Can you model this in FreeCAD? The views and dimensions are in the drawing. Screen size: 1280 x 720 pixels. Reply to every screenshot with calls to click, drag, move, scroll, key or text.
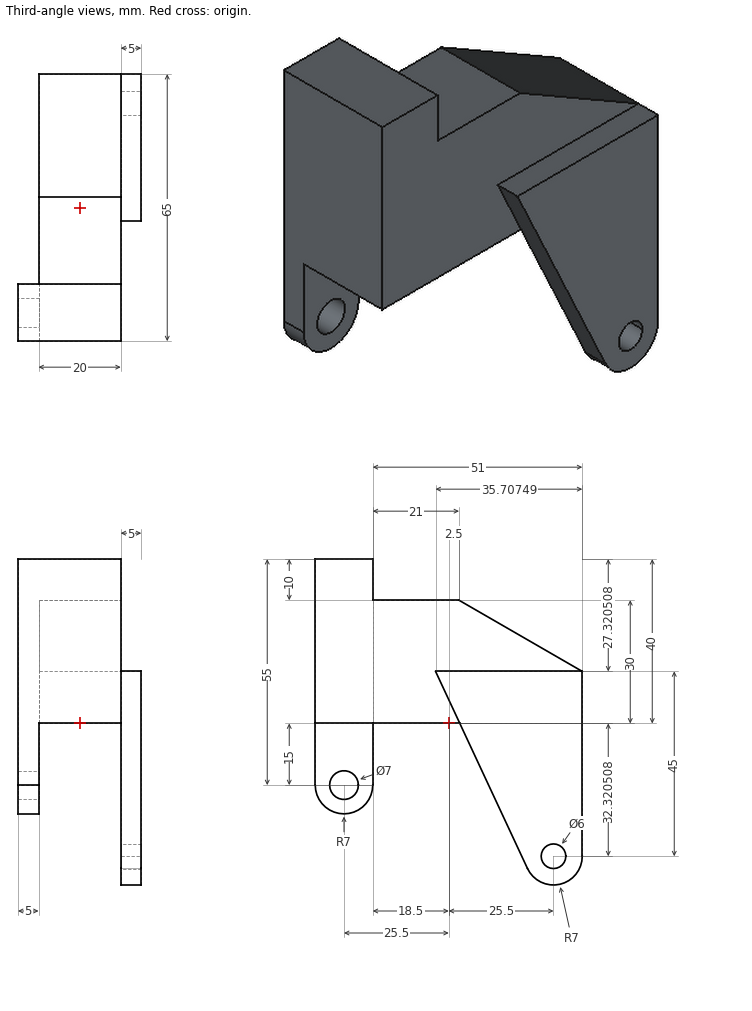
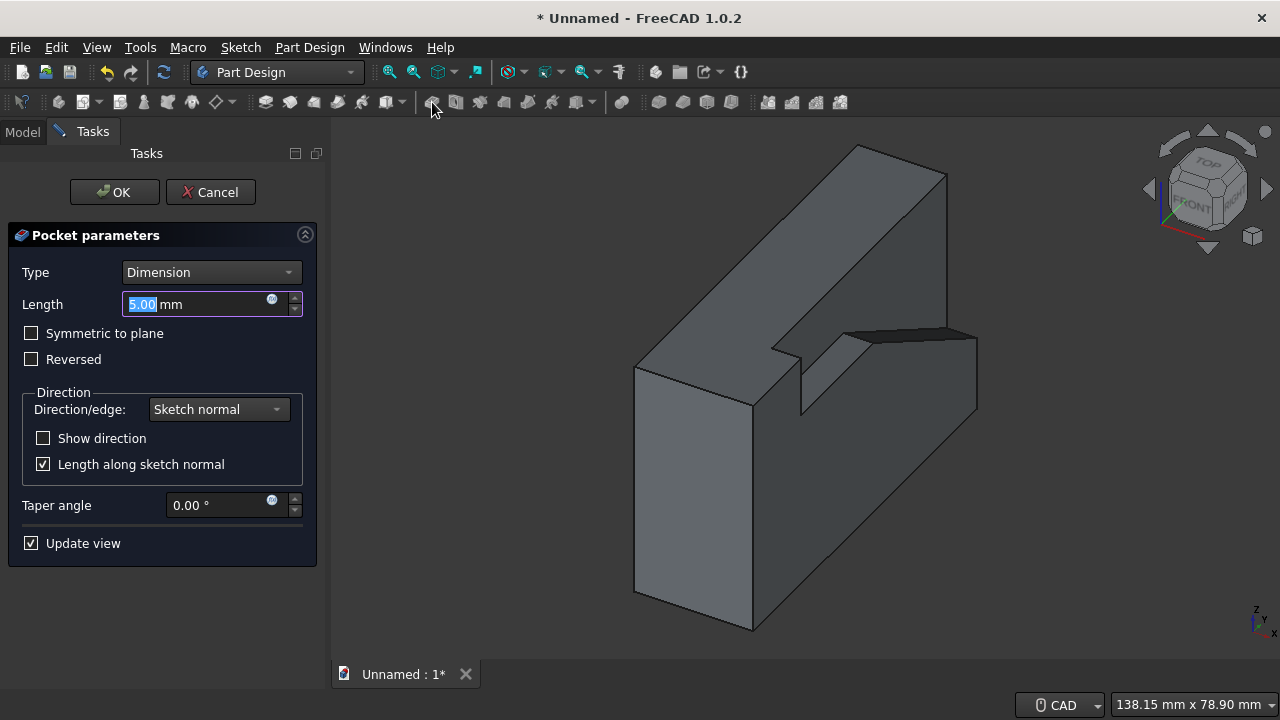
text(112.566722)
key(Tab)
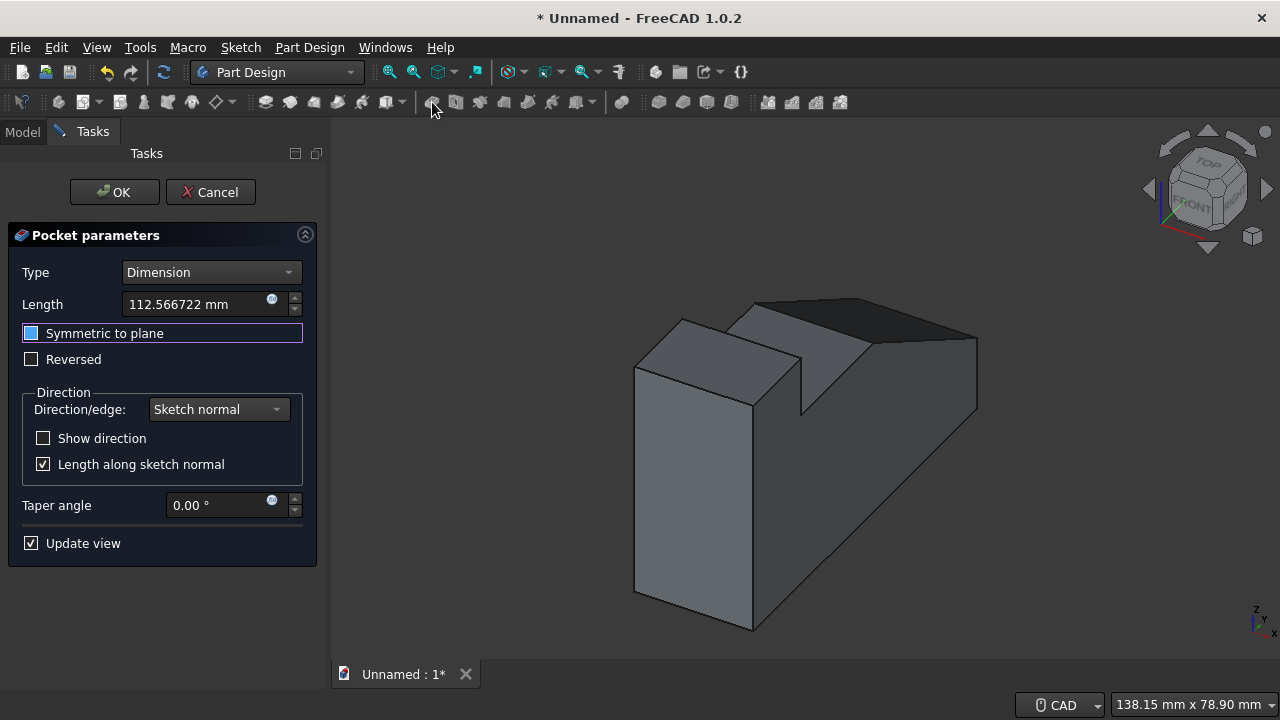
click(30, 333)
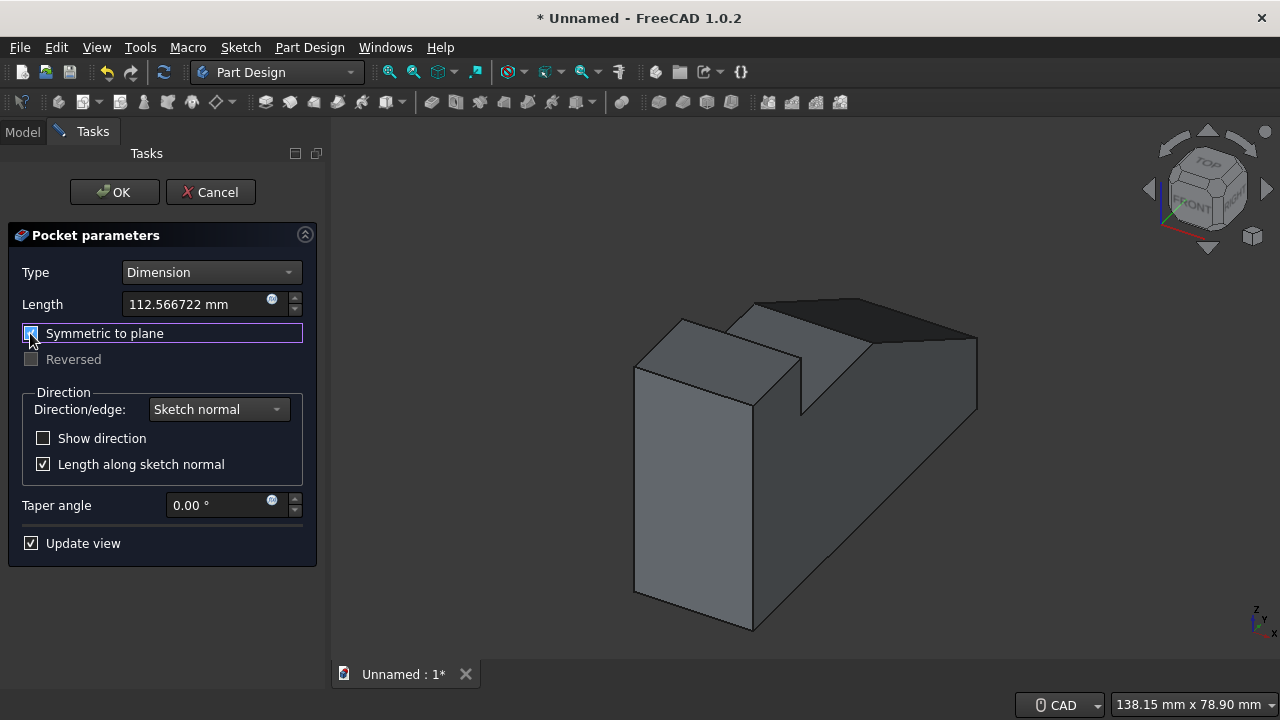
click(115, 192)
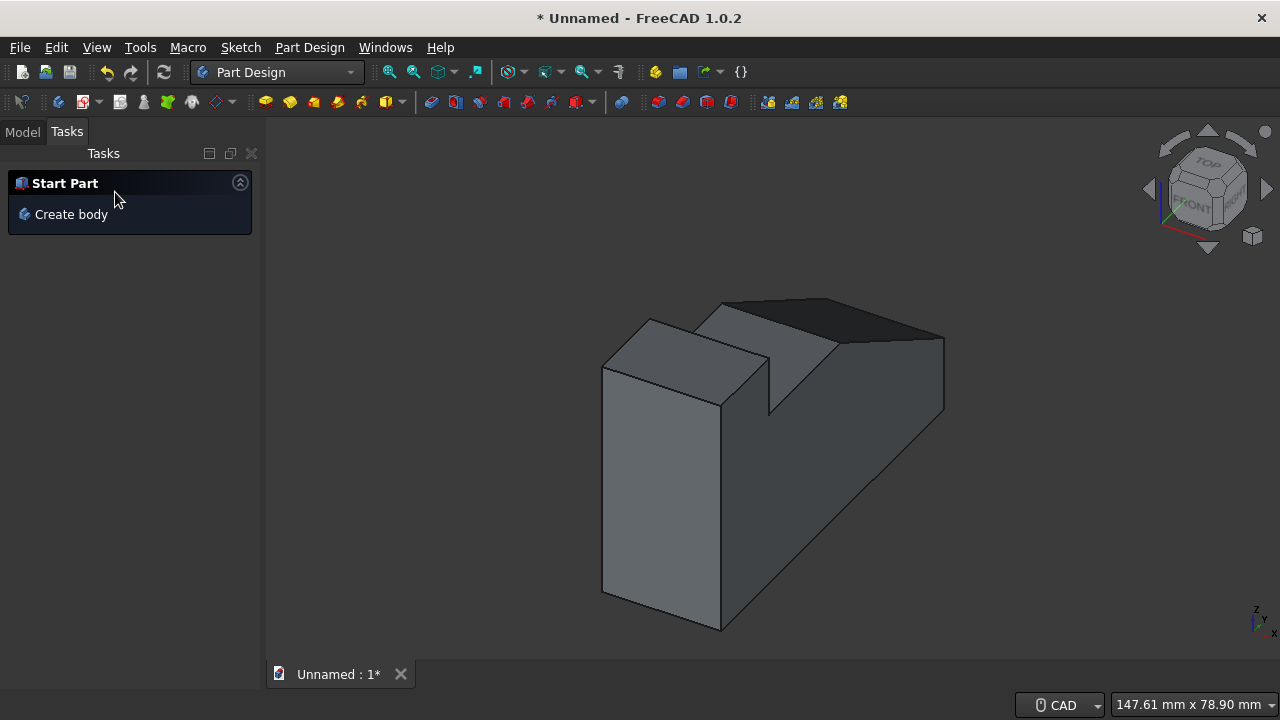
click(832, 439)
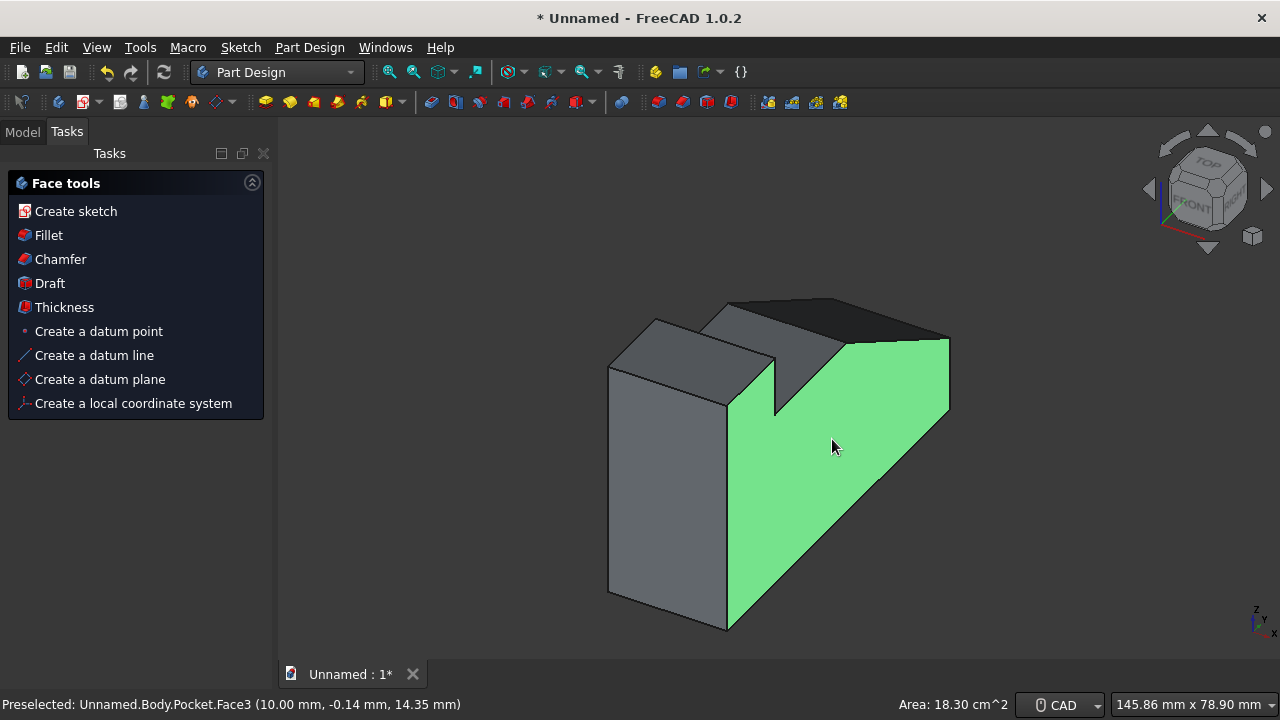
click(84, 102)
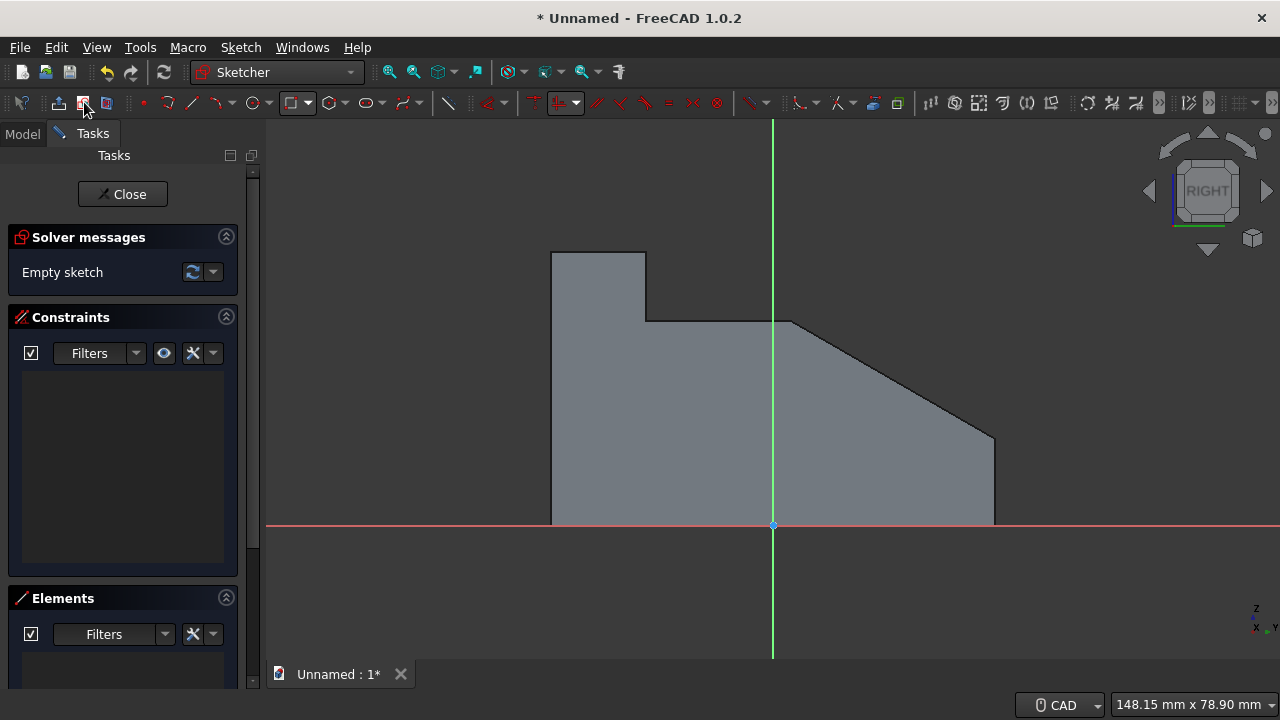
scroll(897, 147, down, 1)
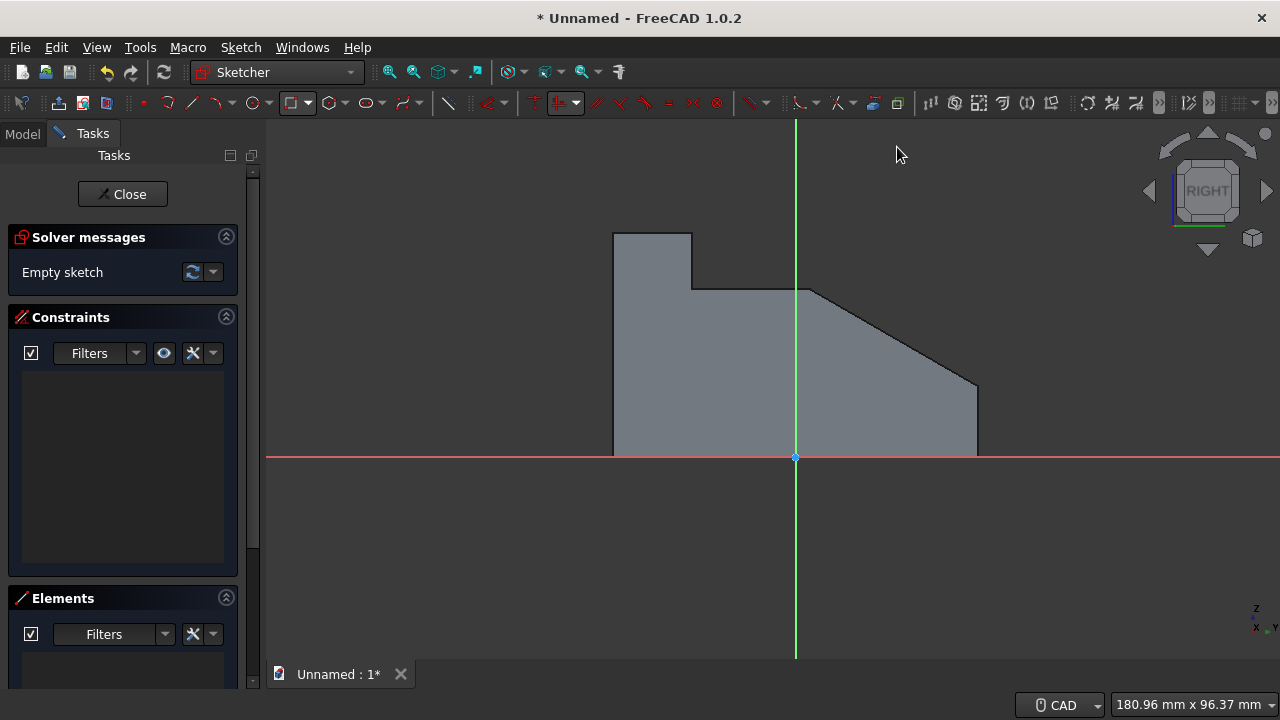
click(168, 104)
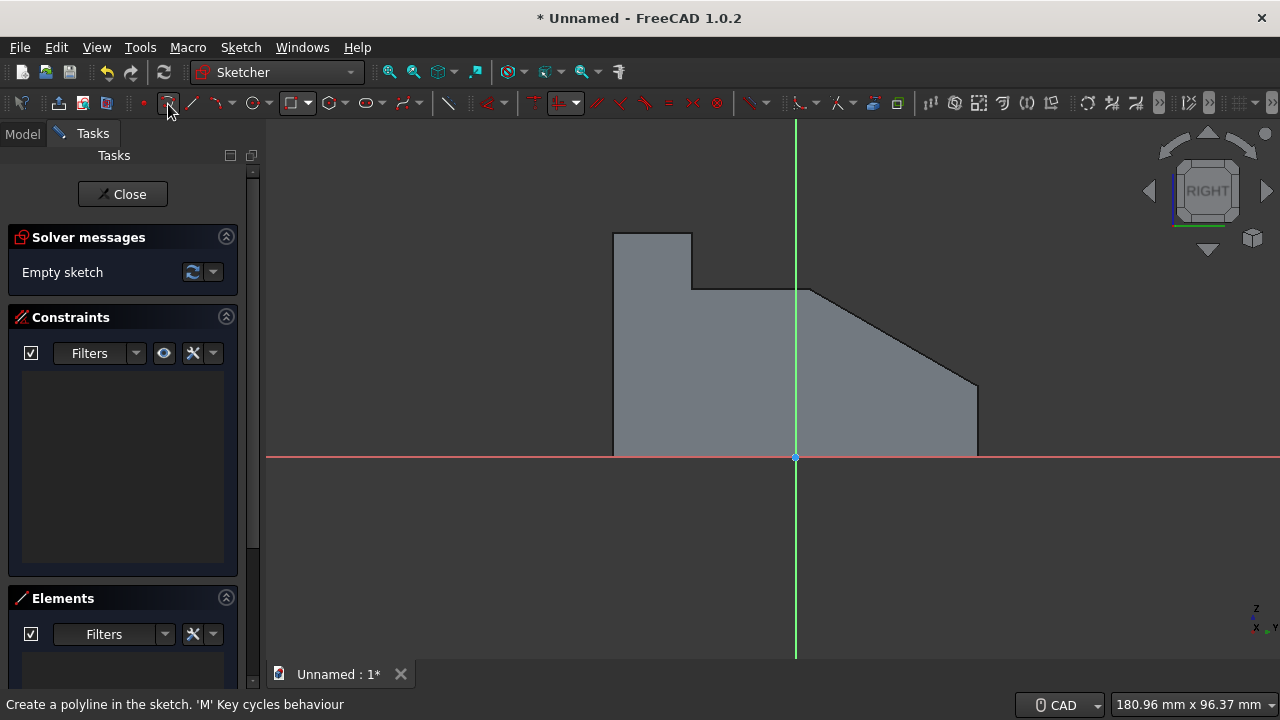
click(692, 541)
click(692, 233)
click(613, 233)
click(613, 541)
right_click(613, 541)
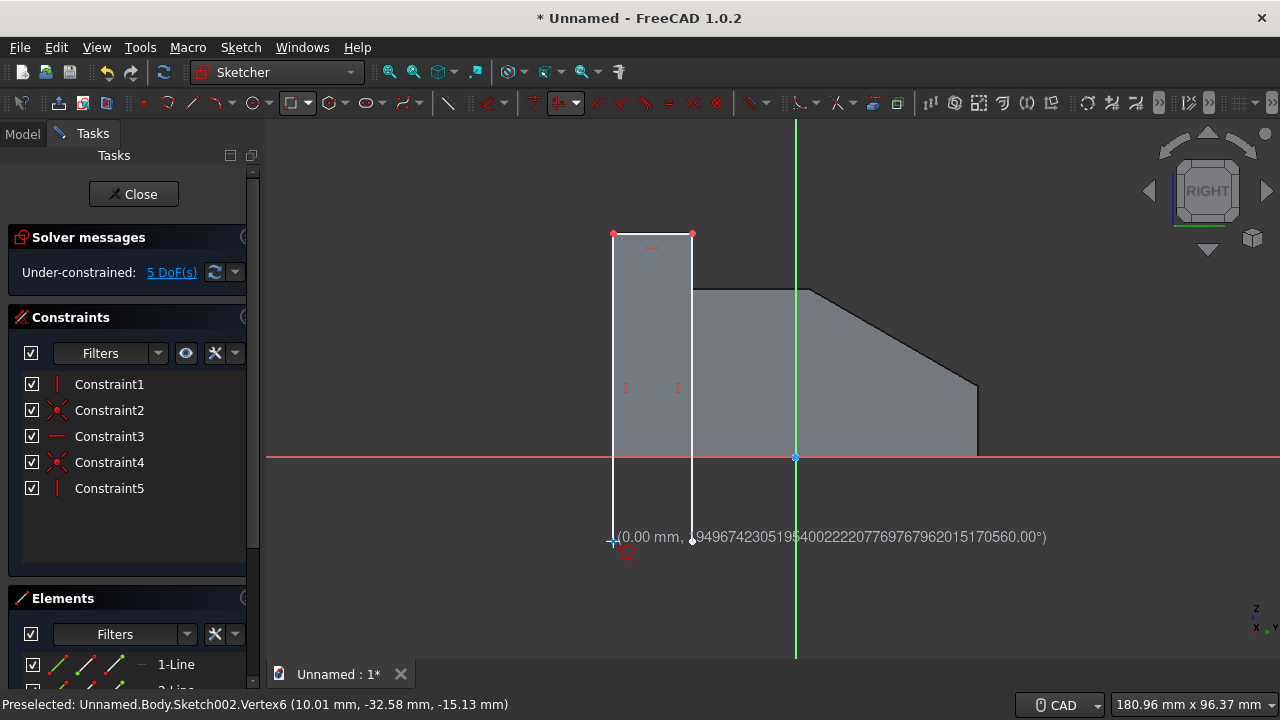
click(216, 104)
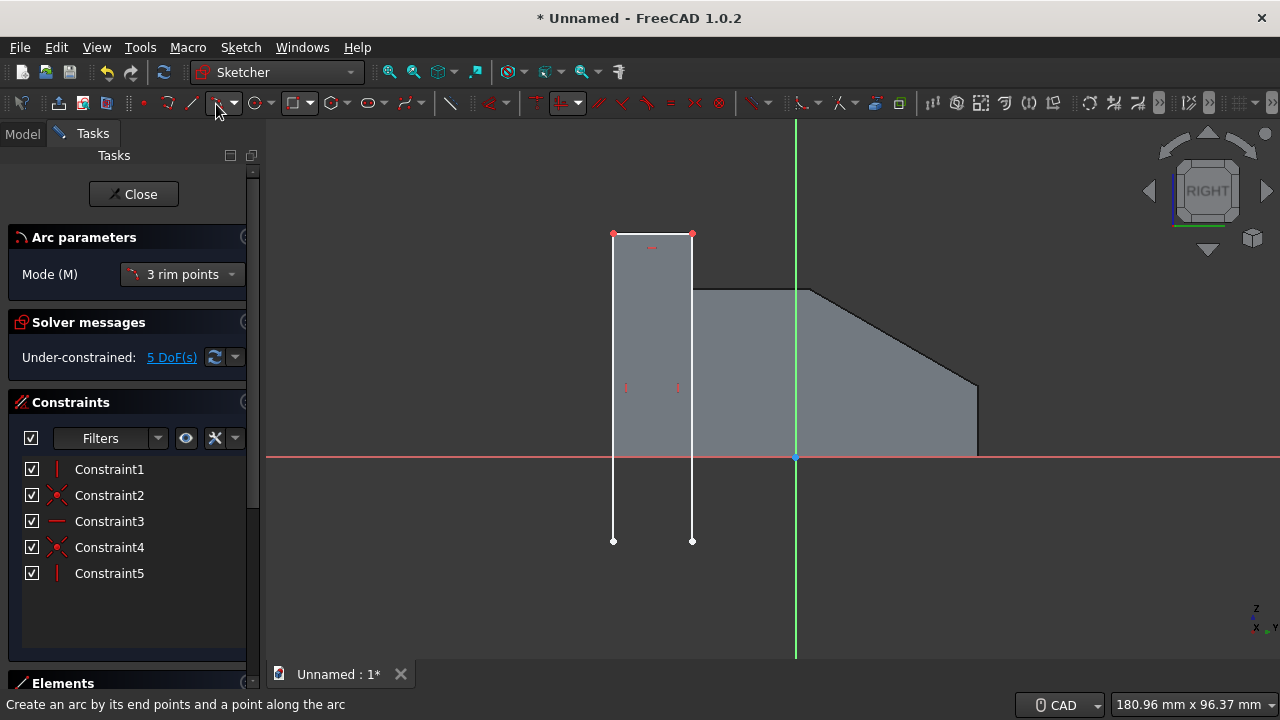
click(613, 542)
click(692, 542)
click(653, 580)
key(Escape)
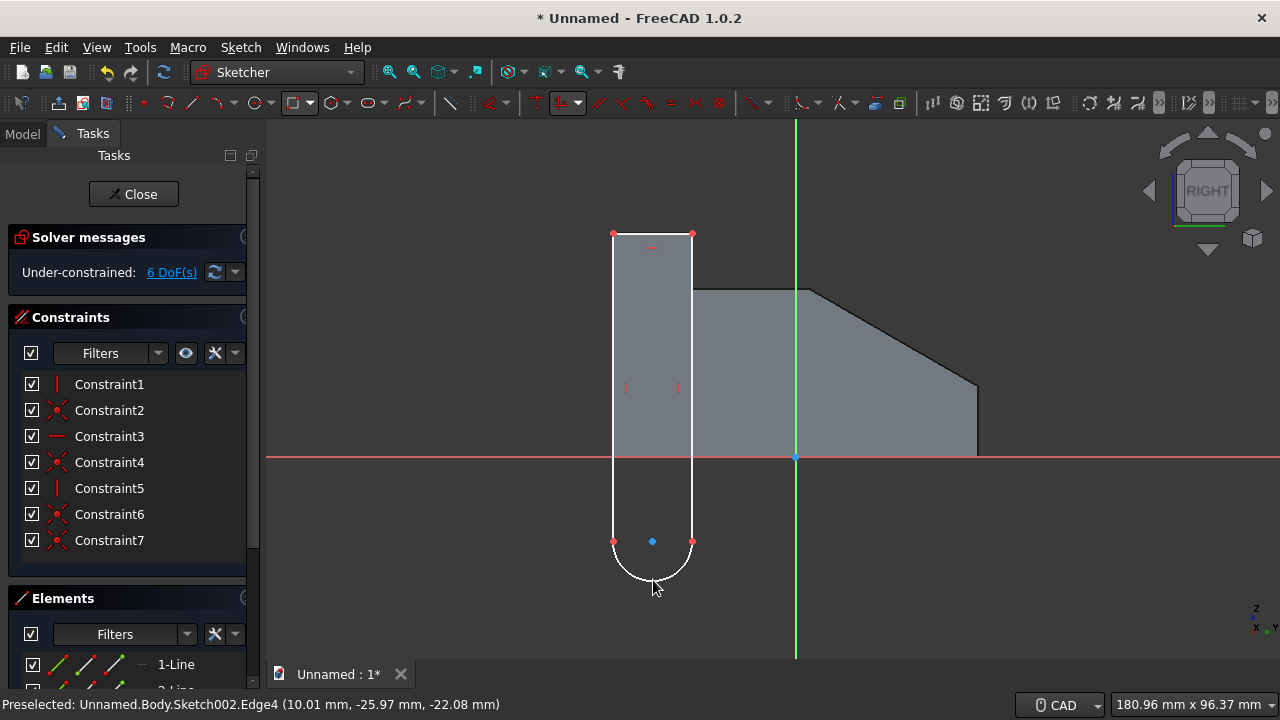
click(692, 326)